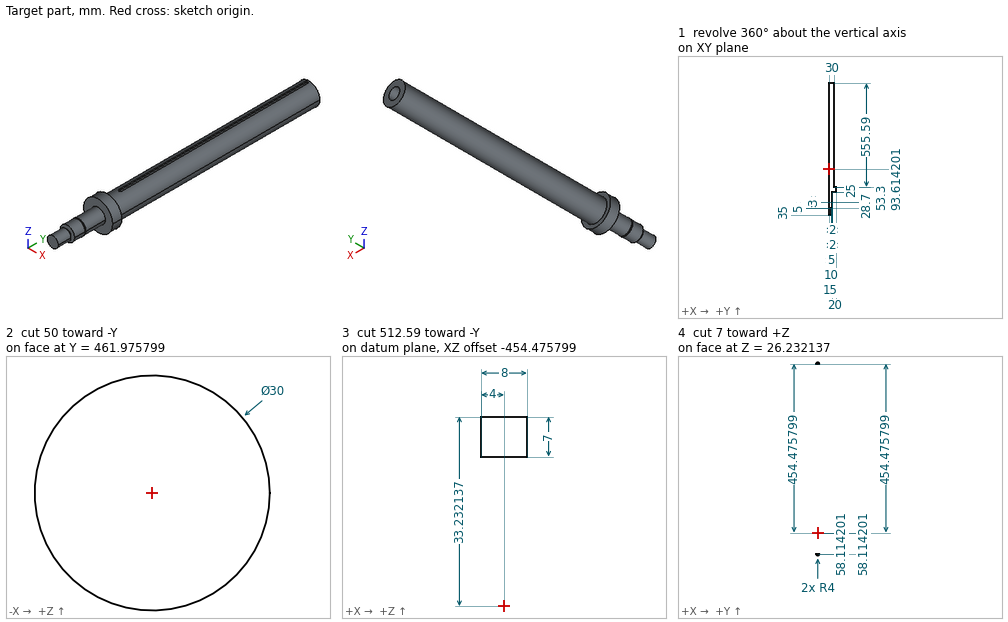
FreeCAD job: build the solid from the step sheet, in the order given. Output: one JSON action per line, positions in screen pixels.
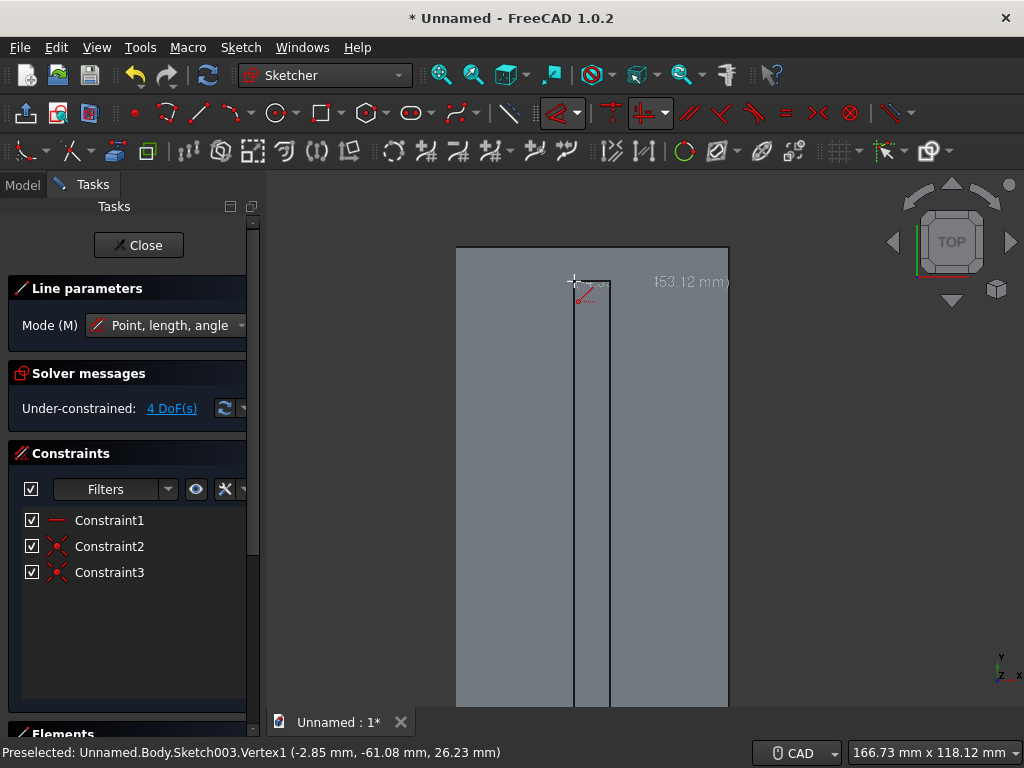
{"action": "left_click", "coordinate": [574, 281]}
{"action": "left_click", "coordinate": [610, 281]}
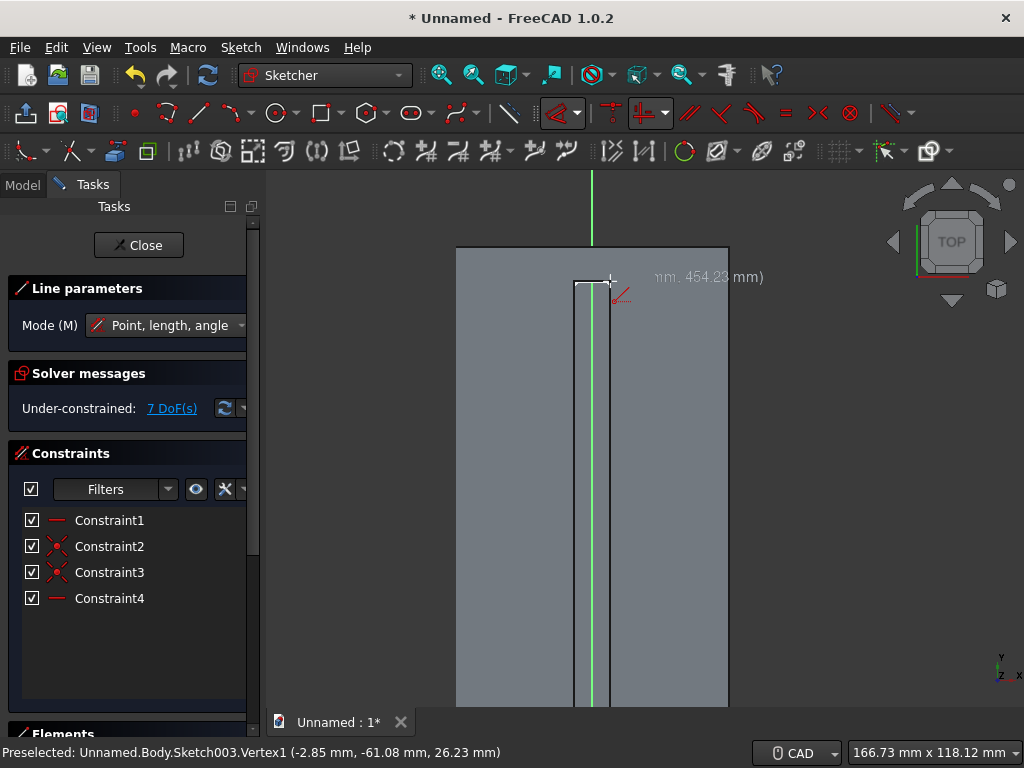
{"action": "key", "text": "g 3 a"}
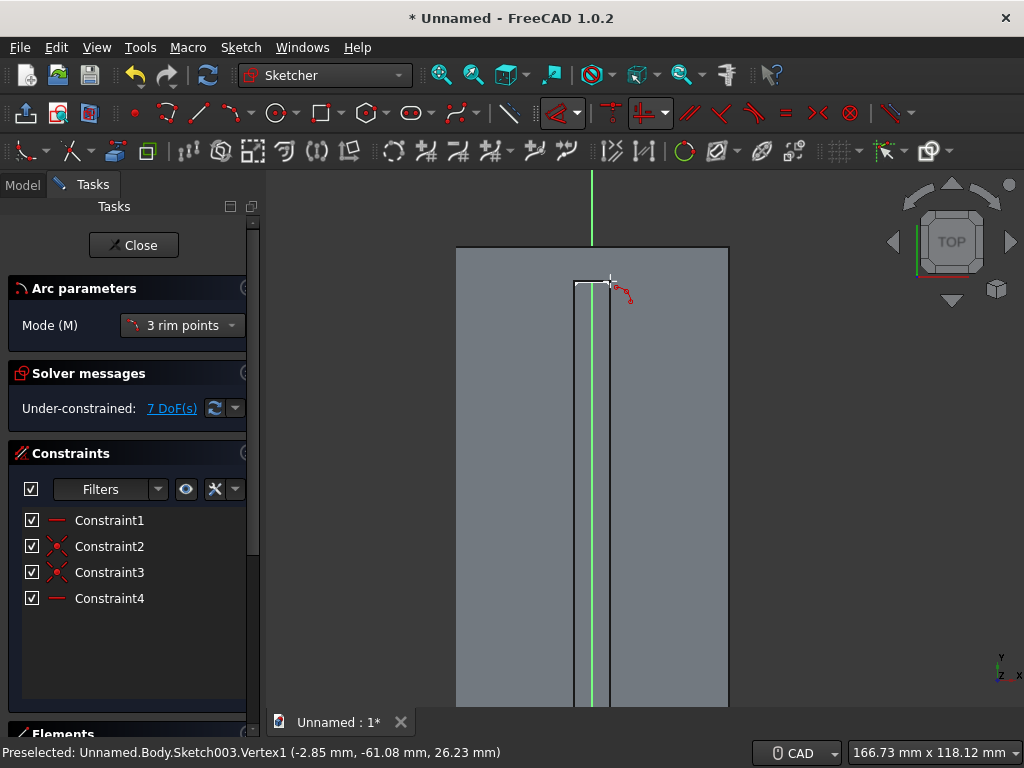
{"action": "left_click", "coordinate": [610, 282]}
{"action": "left_click", "coordinate": [574, 282]}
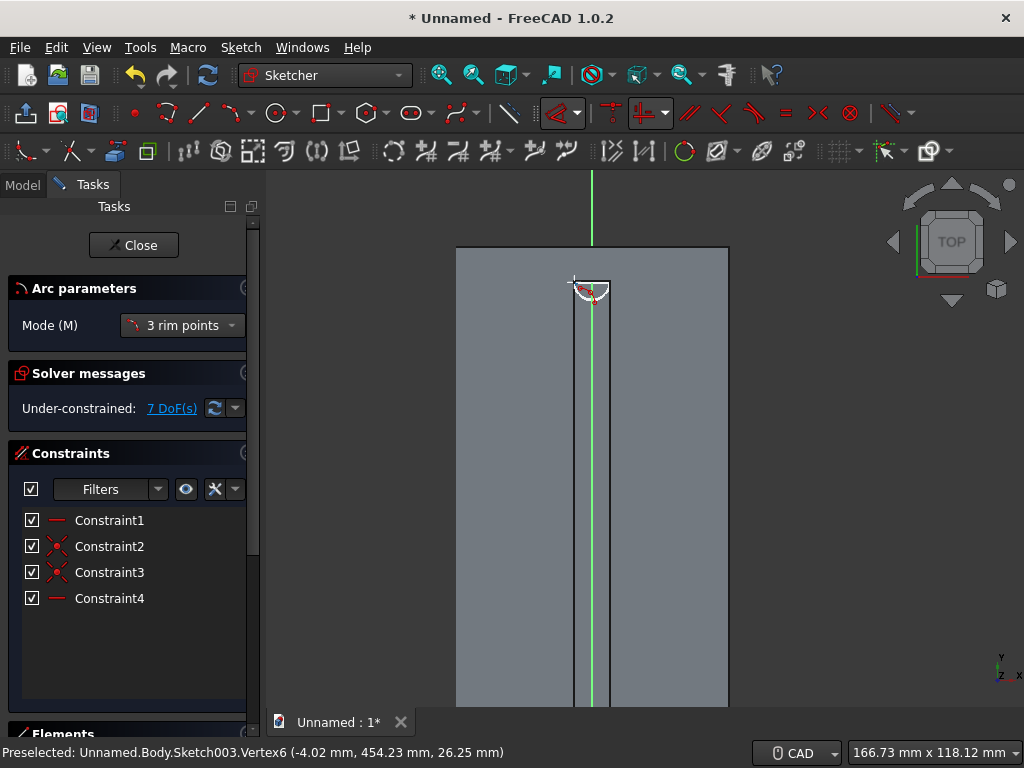
{"action": "scroll", "coordinate": [603, 266], "scroll_direction": "up", "scroll_amount": 2}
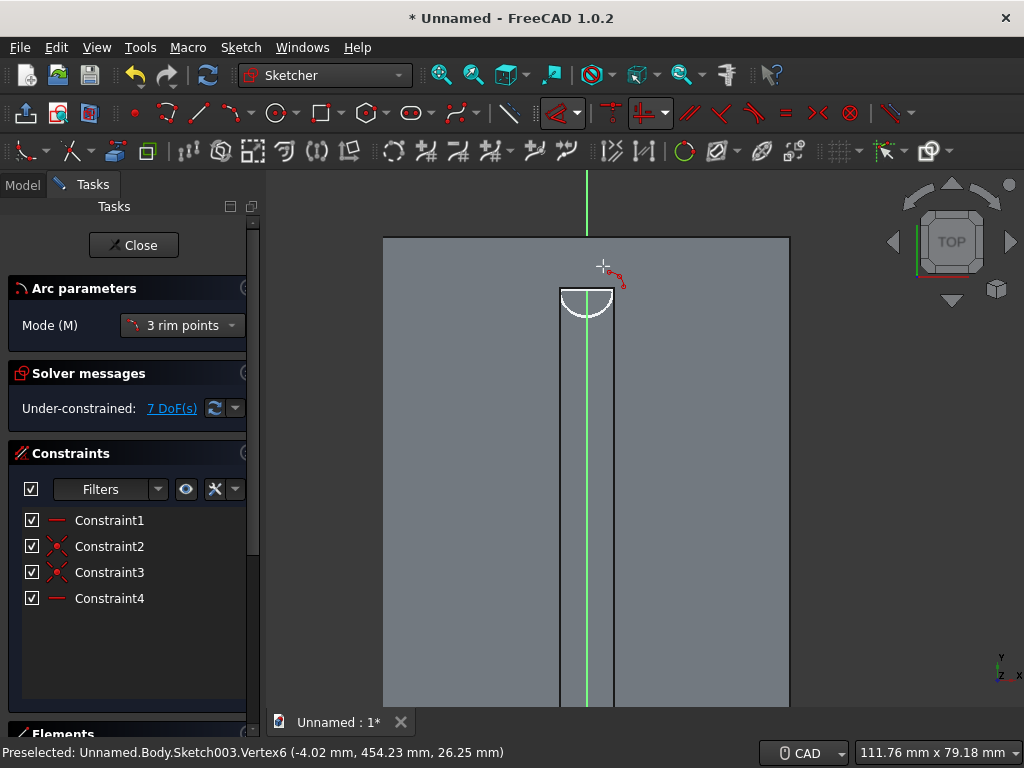
{"action": "left_click", "coordinate": [603, 266]}
{"action": "key", "text": "Escape"}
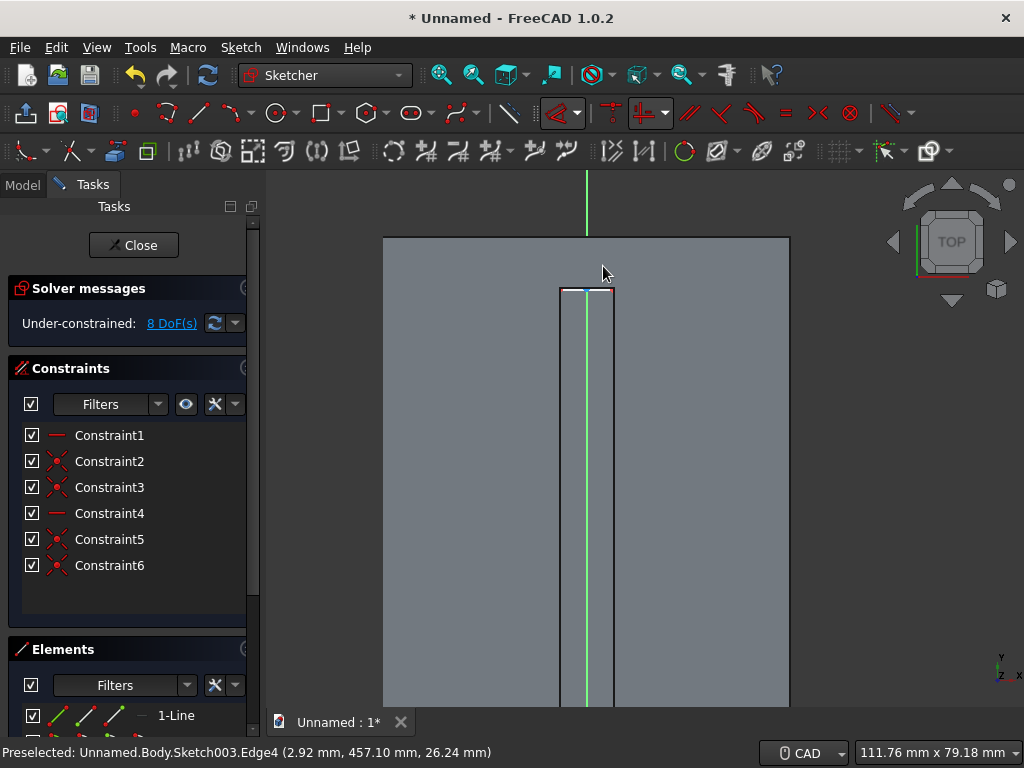
{"action": "scroll", "coordinate": [575, 280], "scroll_direction": "down", "scroll_amount": 12}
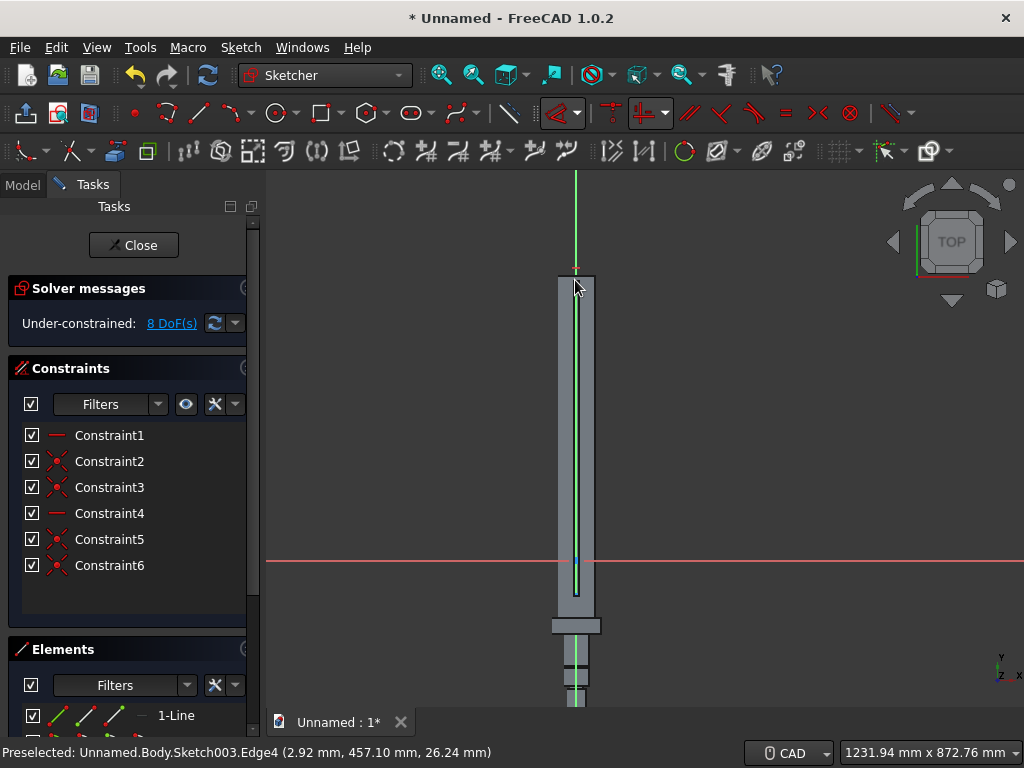
{"action": "scroll", "coordinate": [575, 598], "scroll_direction": "up", "scroll_amount": 12}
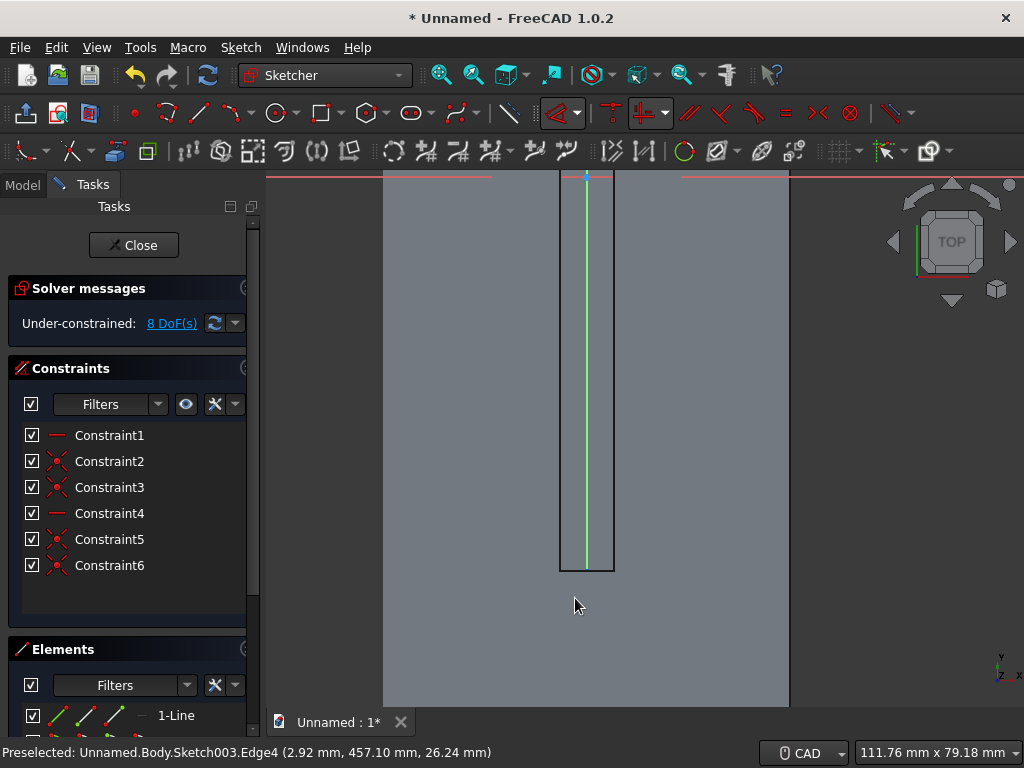
{"action": "left_click", "coordinate": [571, 595]}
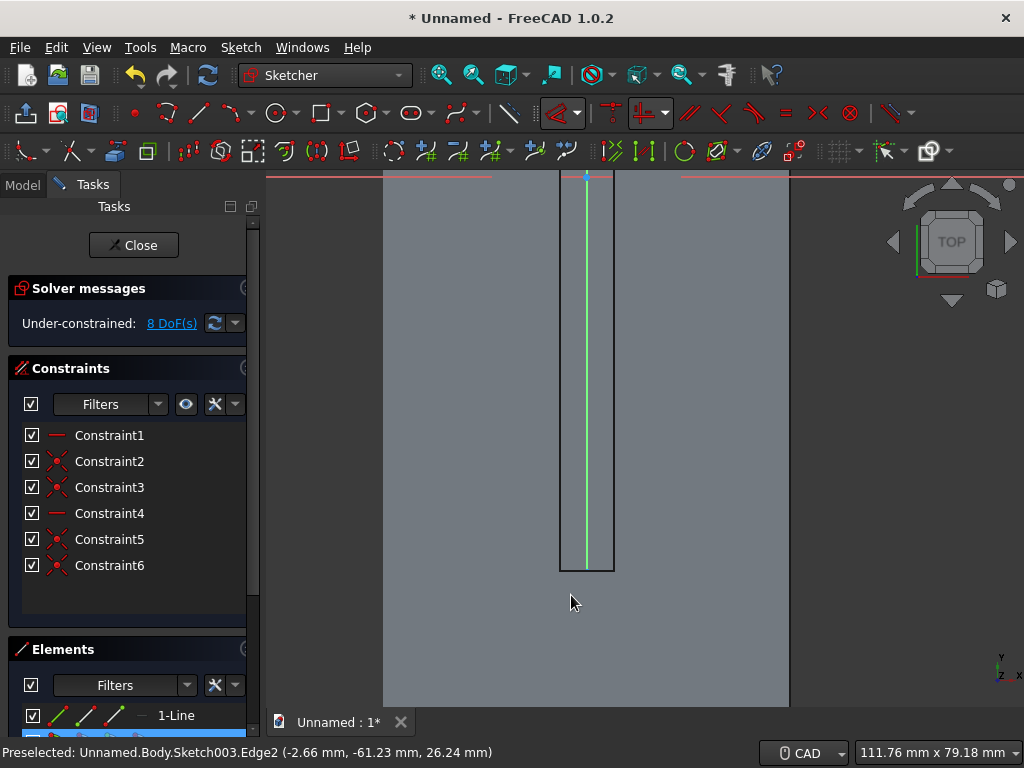
{"action": "scroll", "coordinate": [575, 599], "scroll_direction": "down", "scroll_amount": 12}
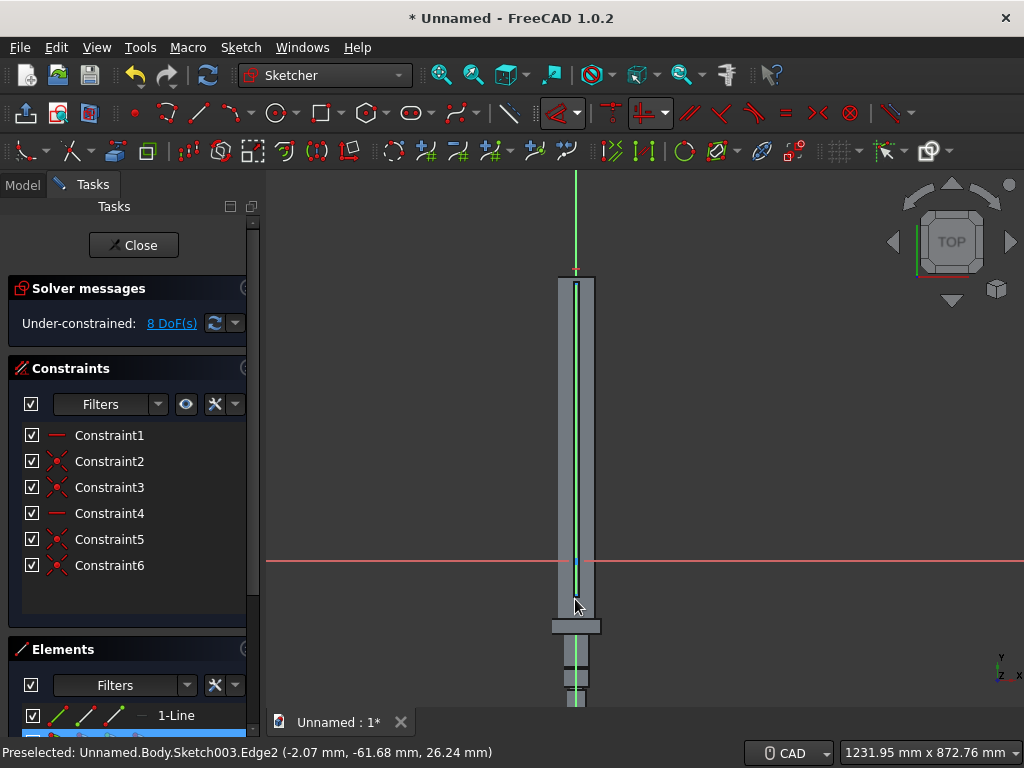
{"action": "scroll", "coordinate": [578, 280], "scroll_direction": "up", "scroll_amount": 12}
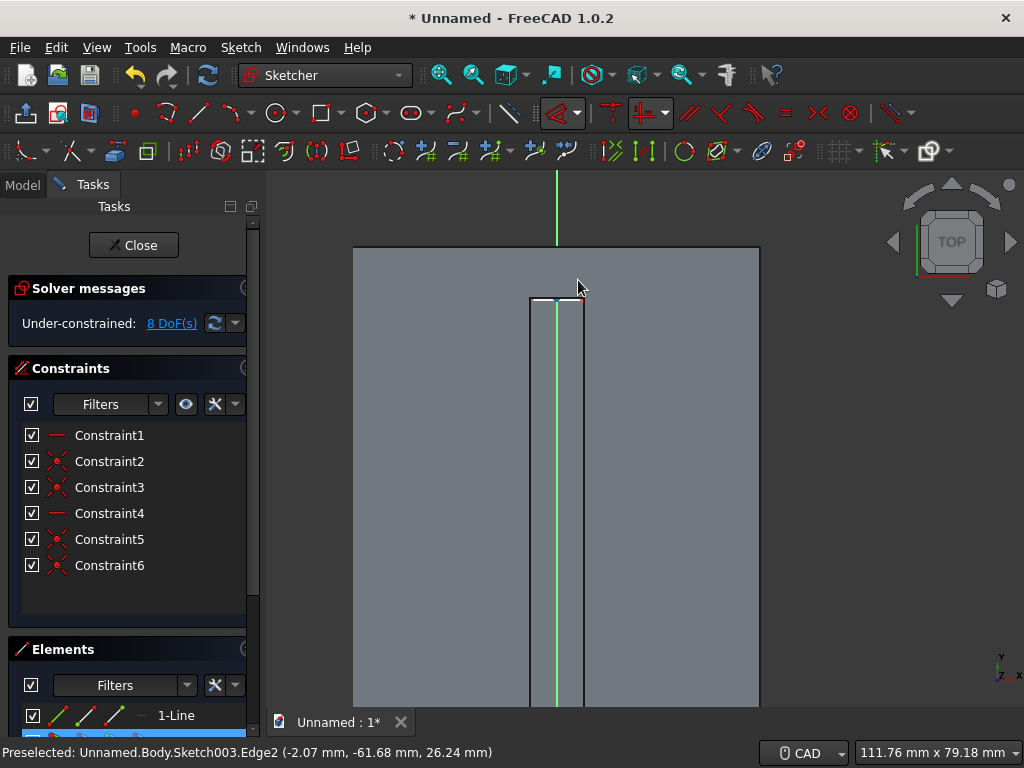
{"action": "left_click", "coordinate": [573, 277]}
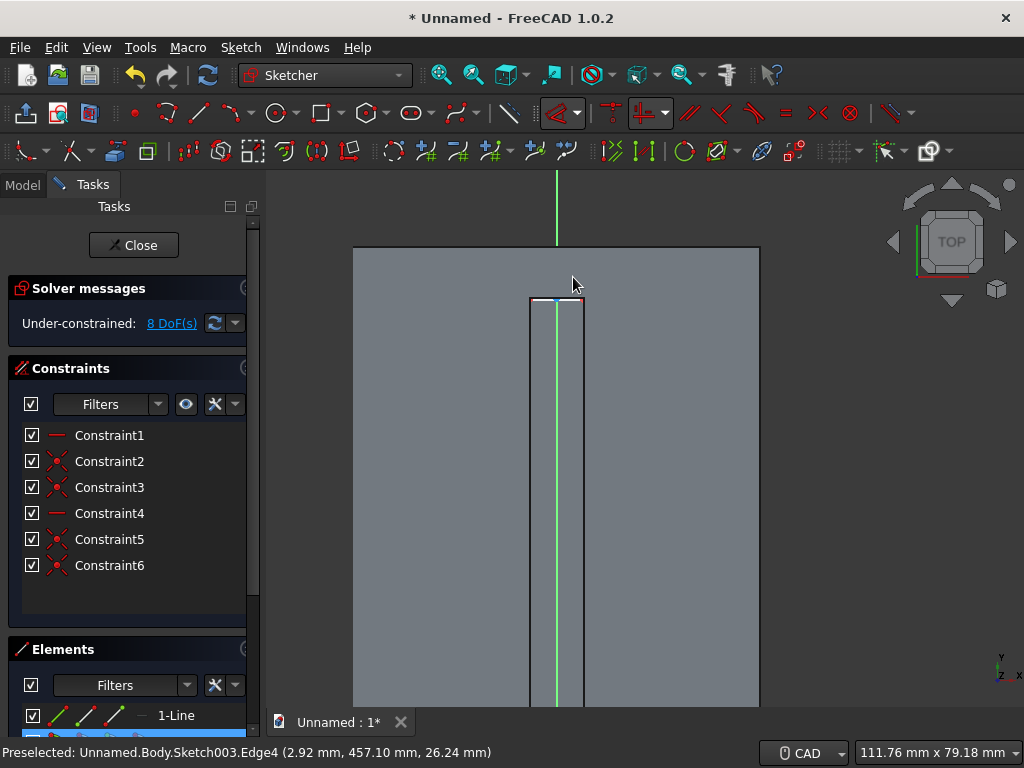
{"action": "key", "text": "e"}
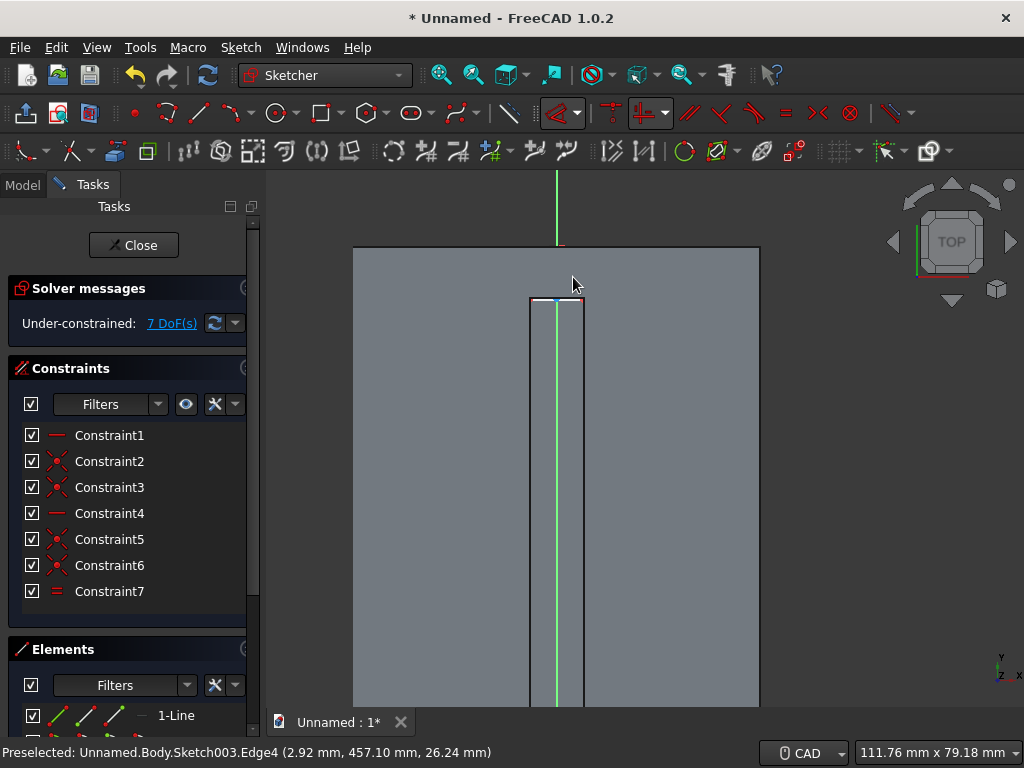
{"action": "scroll", "coordinate": [578, 279], "scroll_direction": "down", "scroll_amount": 12}